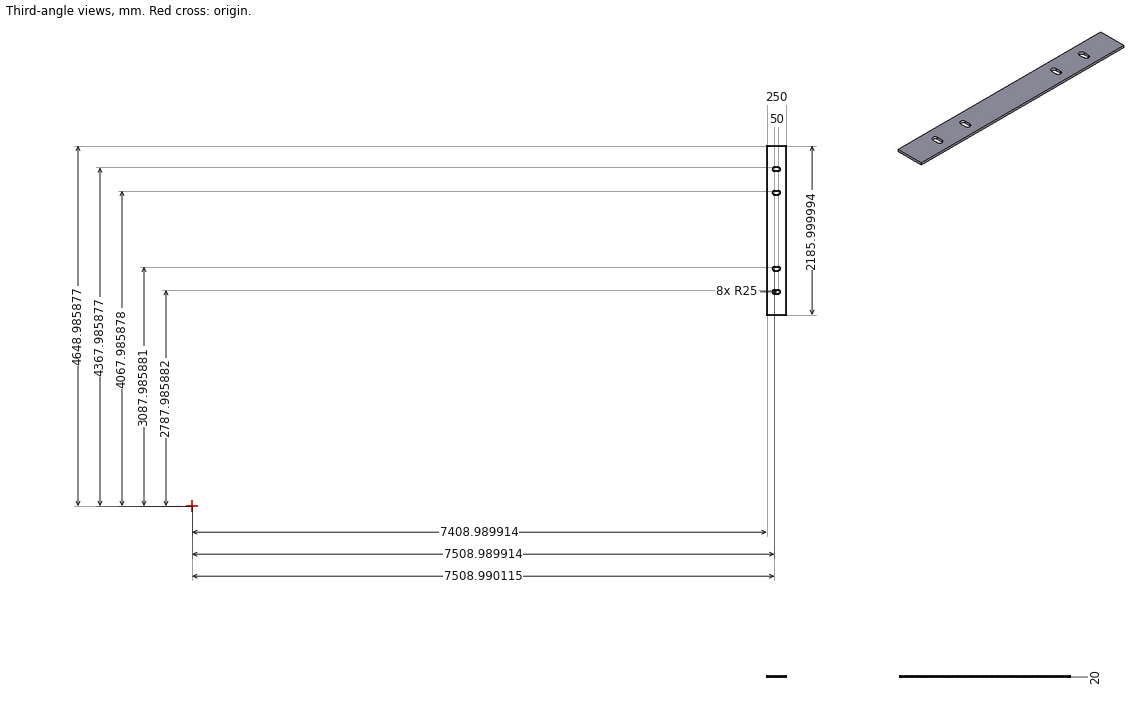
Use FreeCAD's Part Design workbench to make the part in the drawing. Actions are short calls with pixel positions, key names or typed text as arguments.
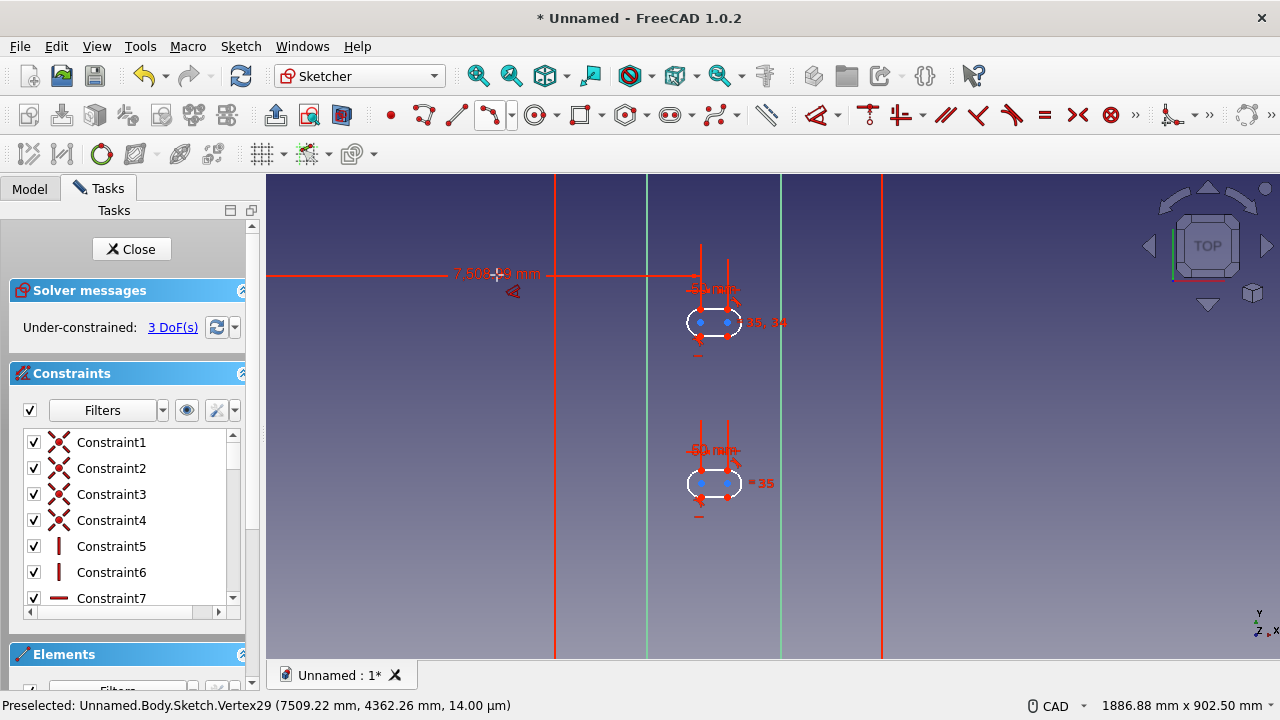
click(701, 309)
click(735, 396)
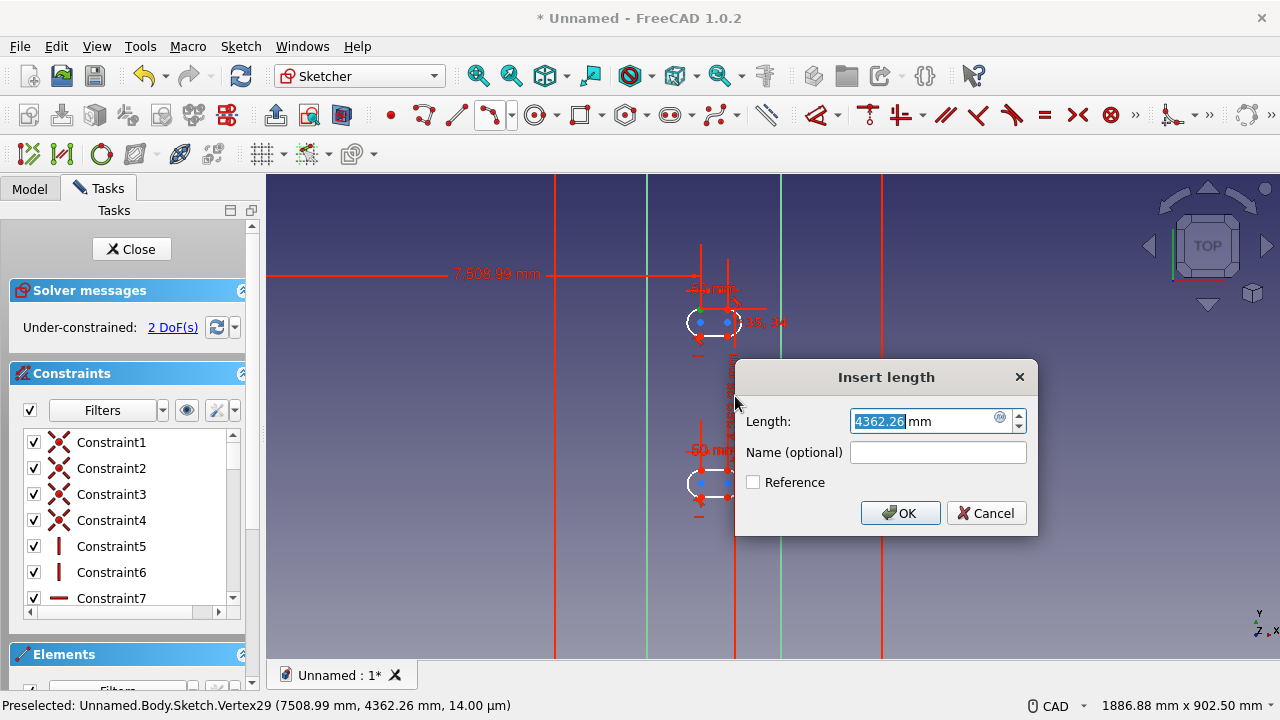
text(4367.985877)
key(Return)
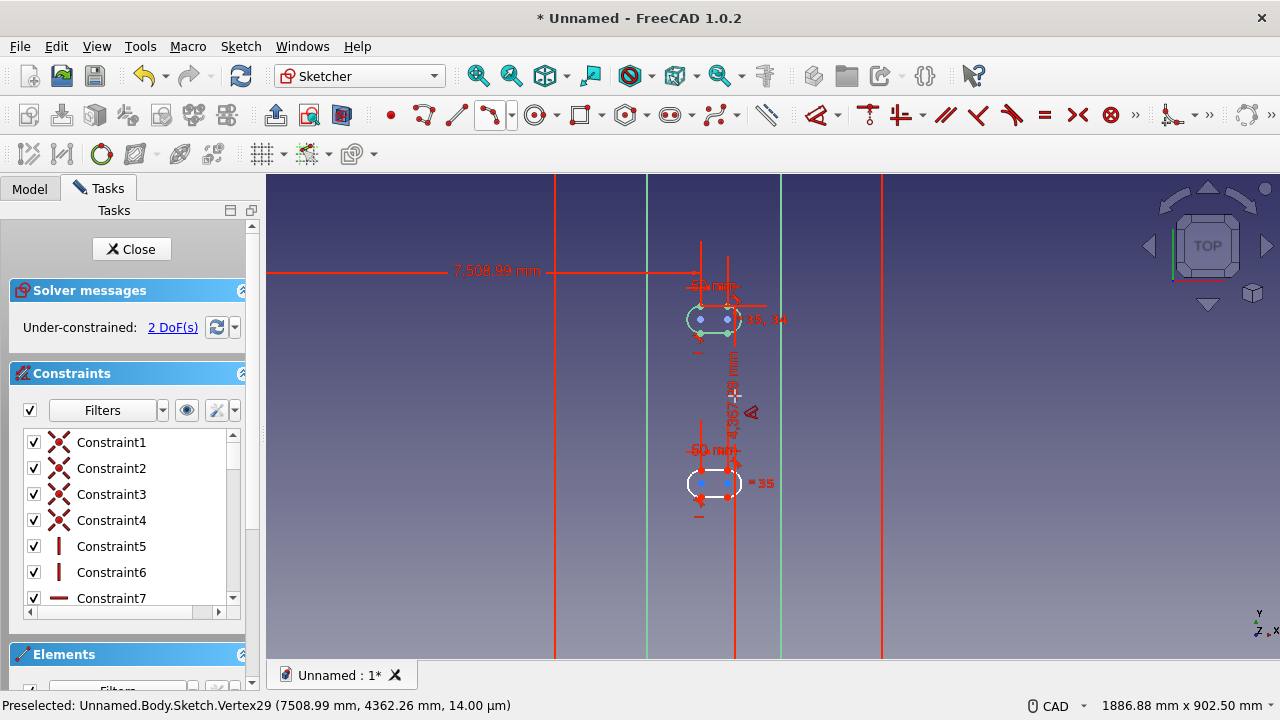
click(701, 470)
click(498, 436)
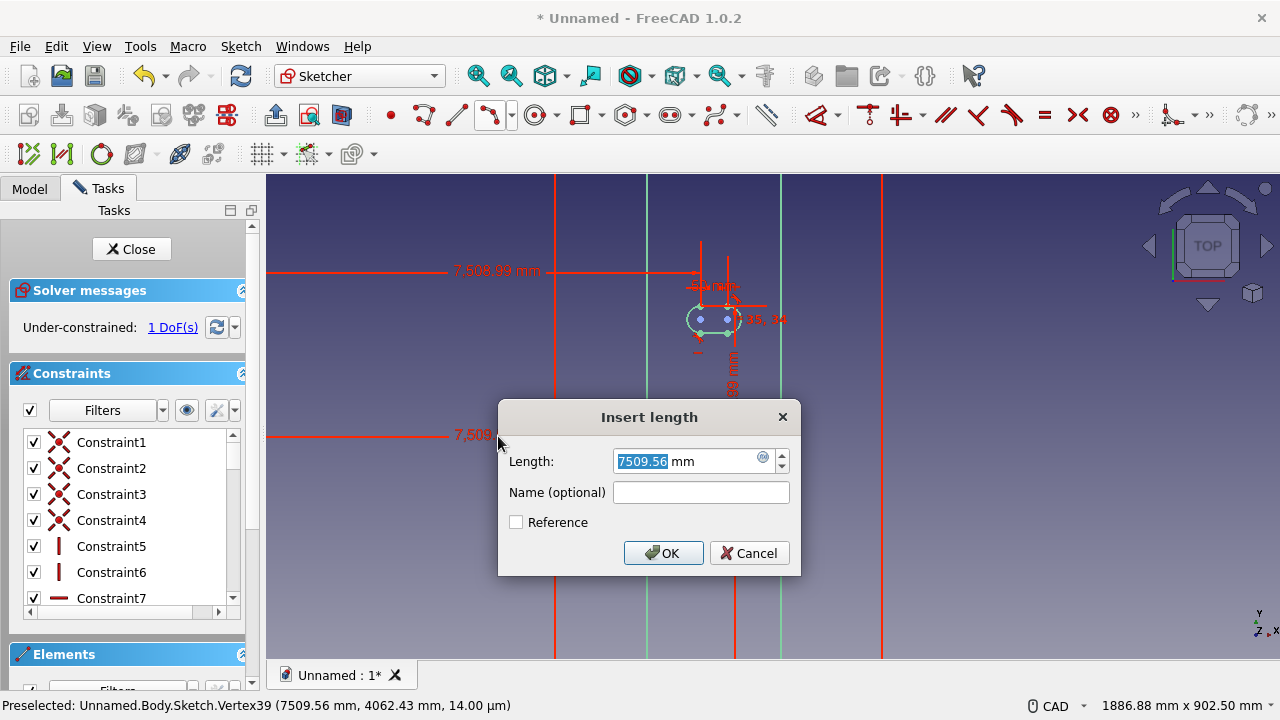
text(7508.989914)
key(Return)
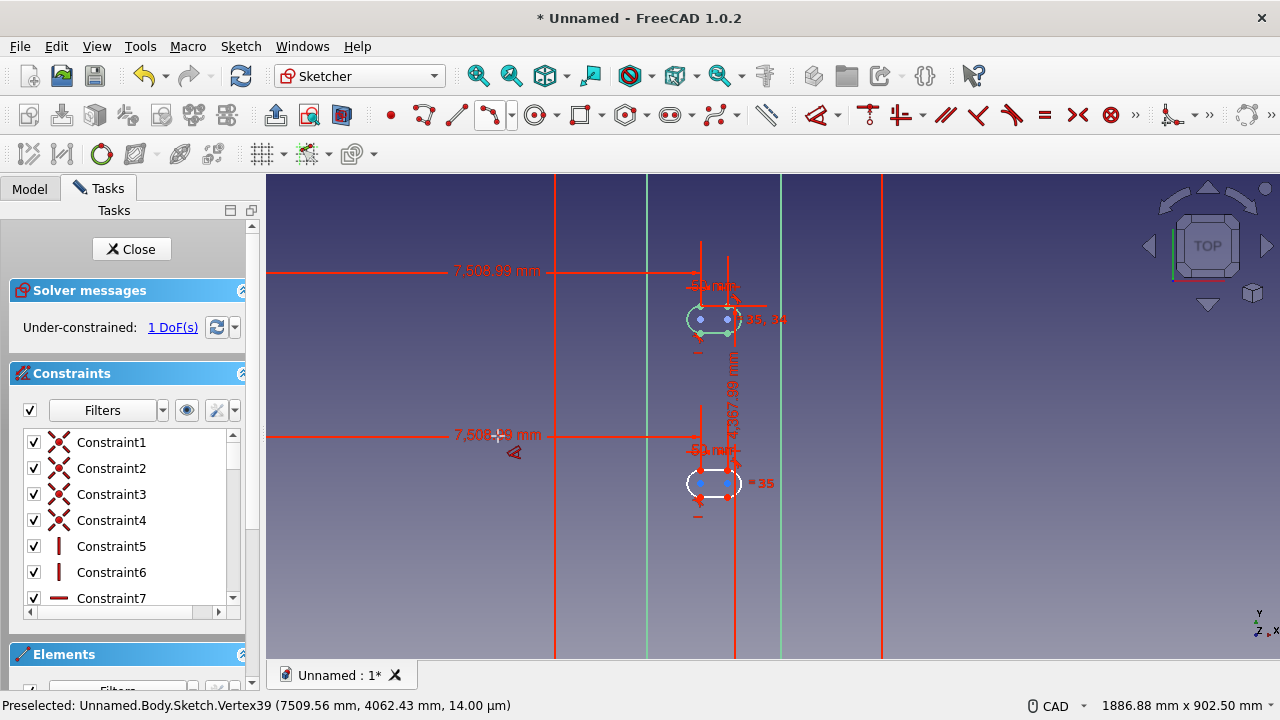
click(701, 470)
click(735, 551)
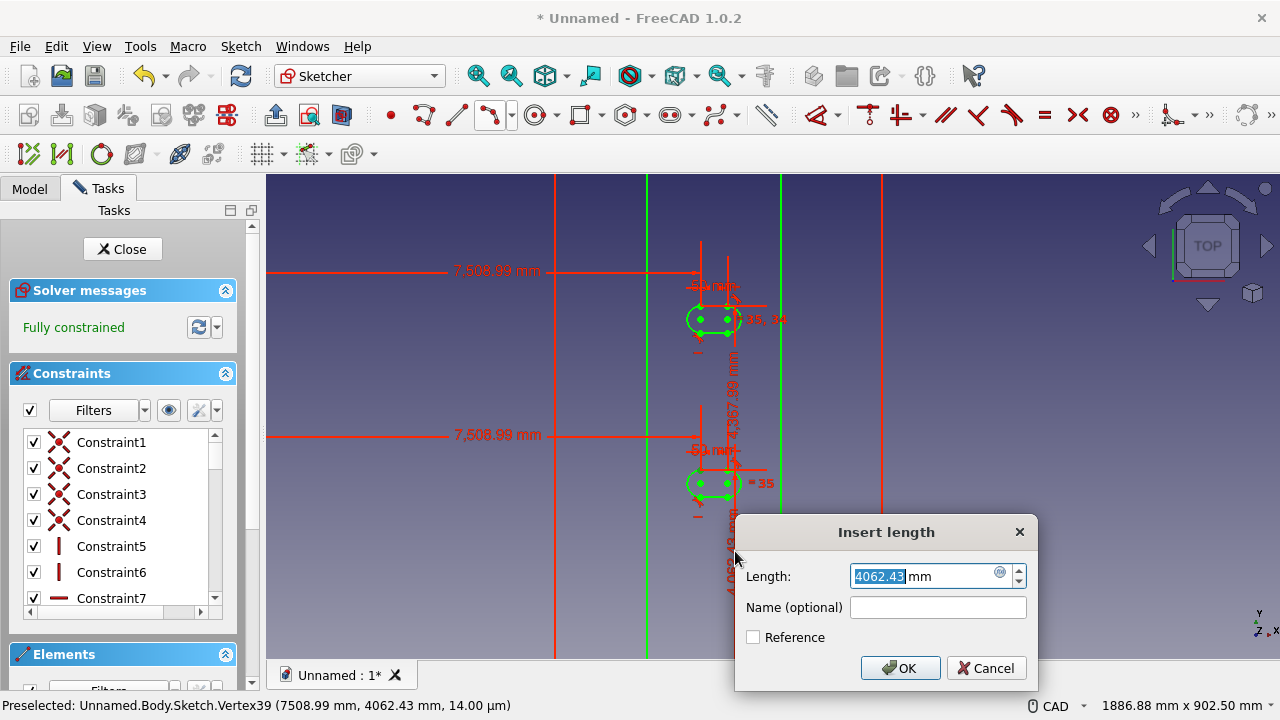
text(4067.985878)
key(Return)
key(Escape)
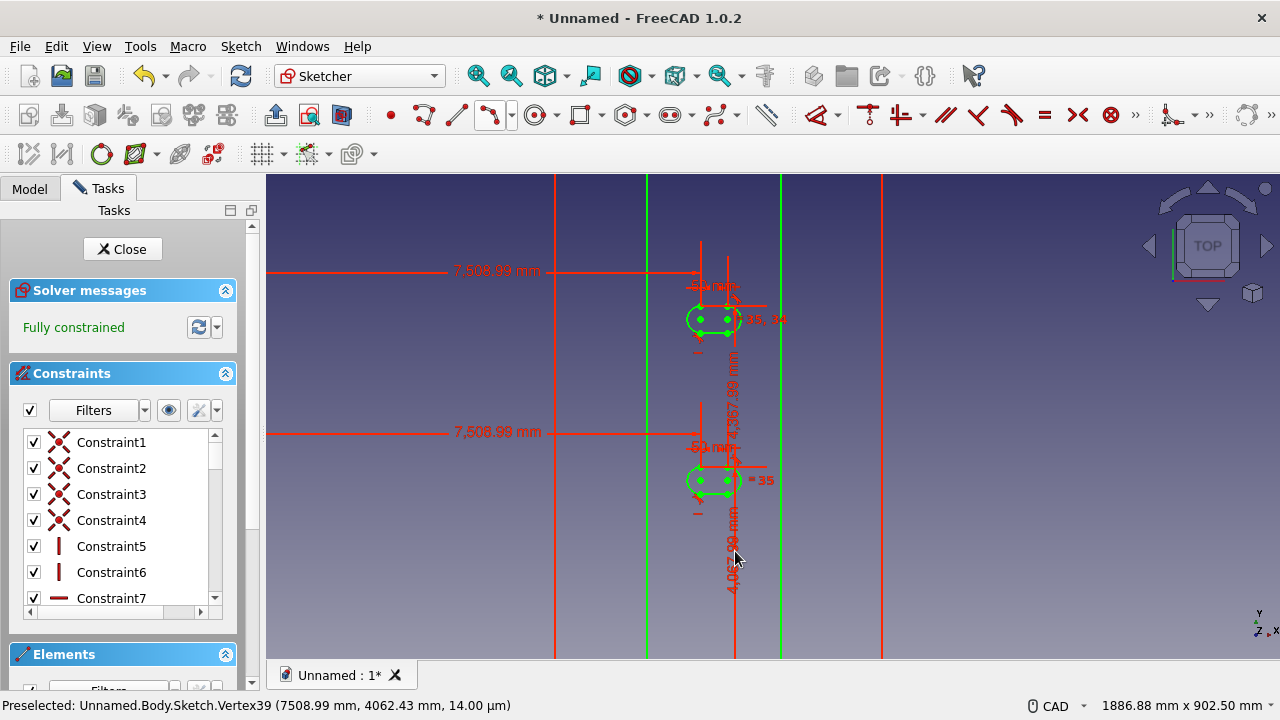
click(123, 249)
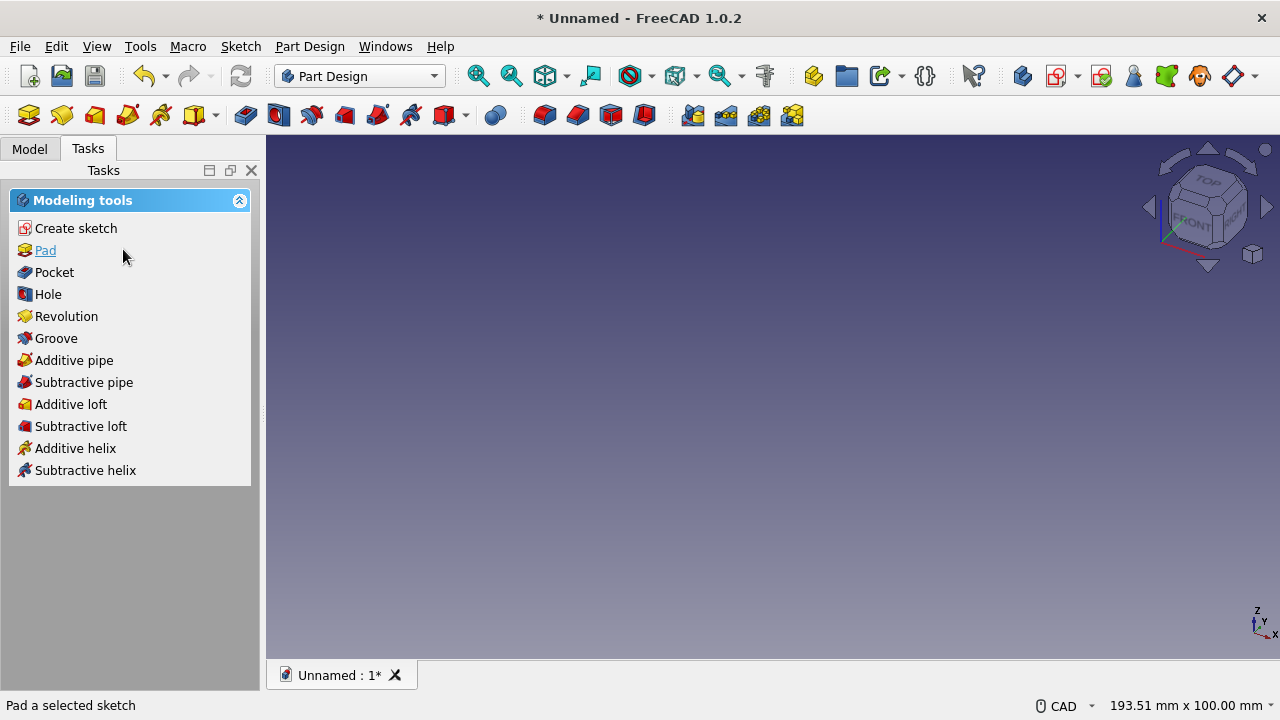
click(29, 116)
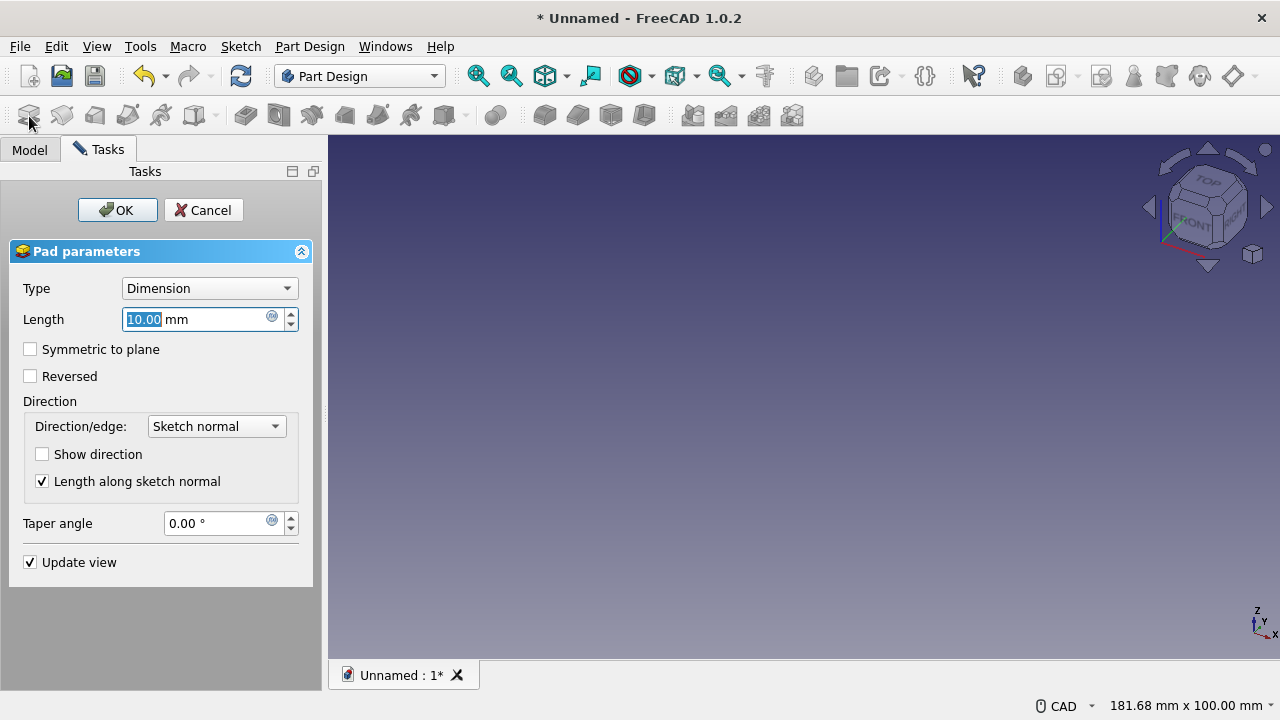
text(20)
key(Tab)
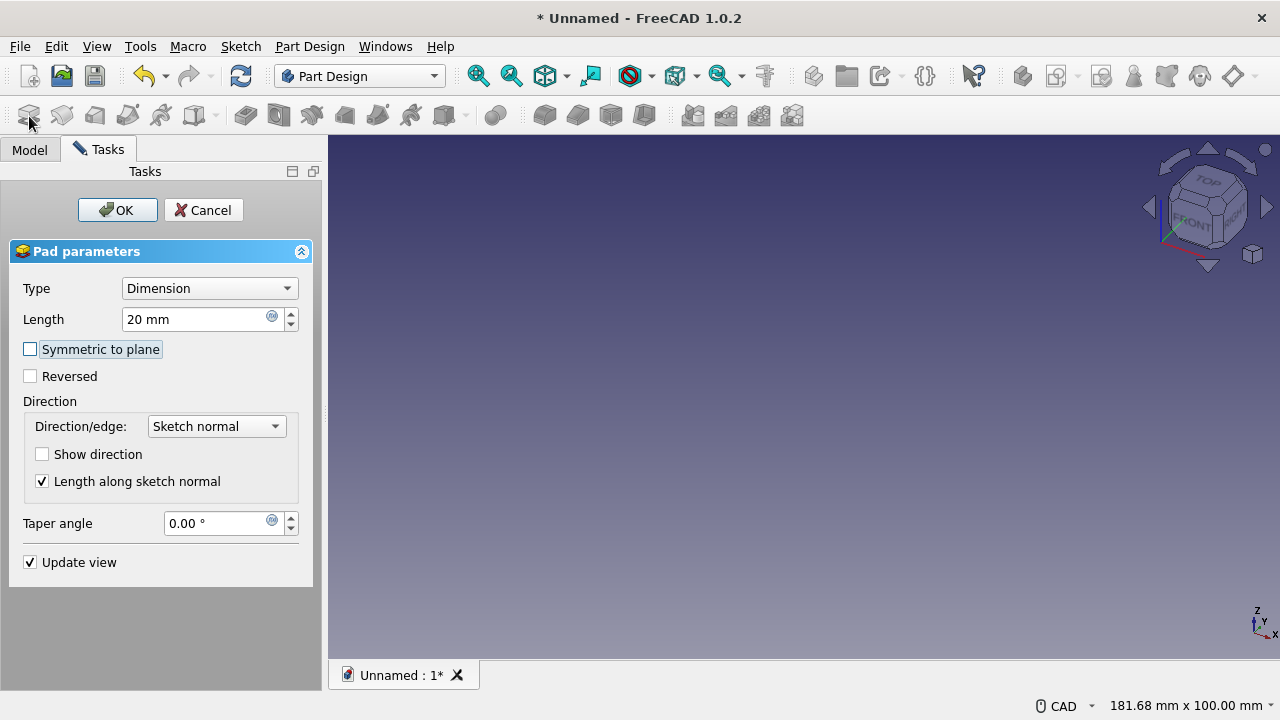
click(118, 210)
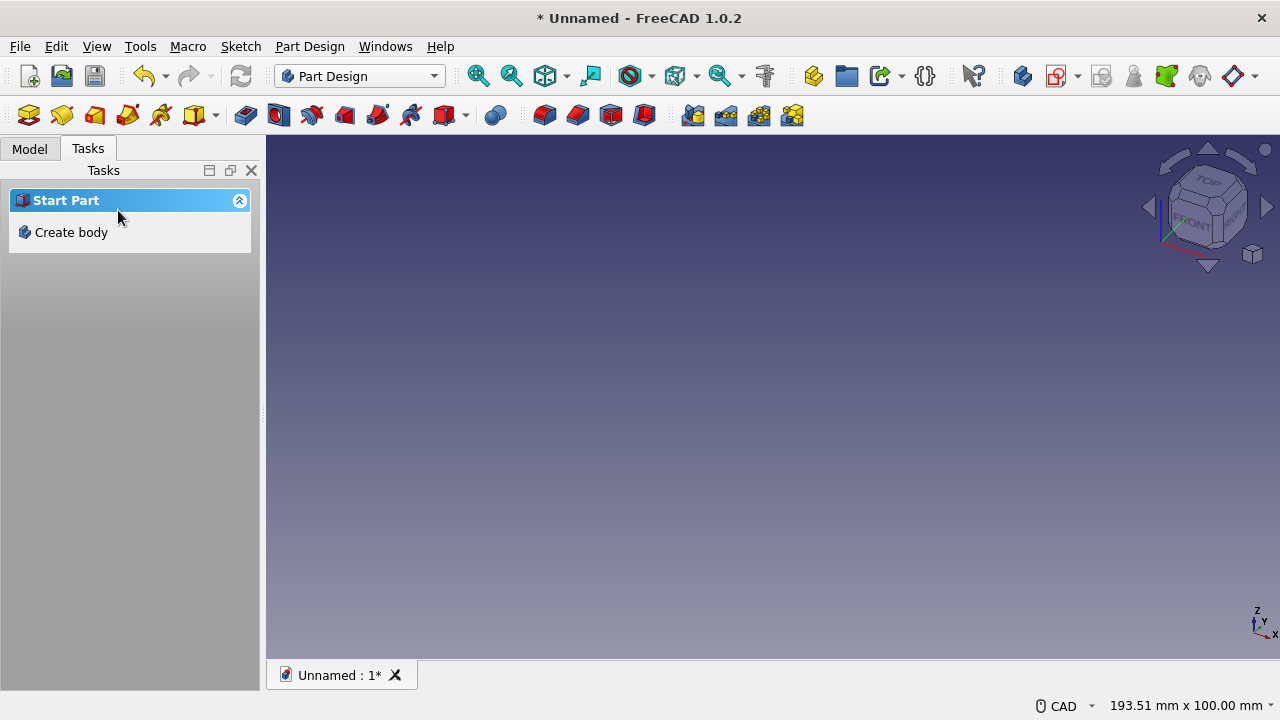
key(0)